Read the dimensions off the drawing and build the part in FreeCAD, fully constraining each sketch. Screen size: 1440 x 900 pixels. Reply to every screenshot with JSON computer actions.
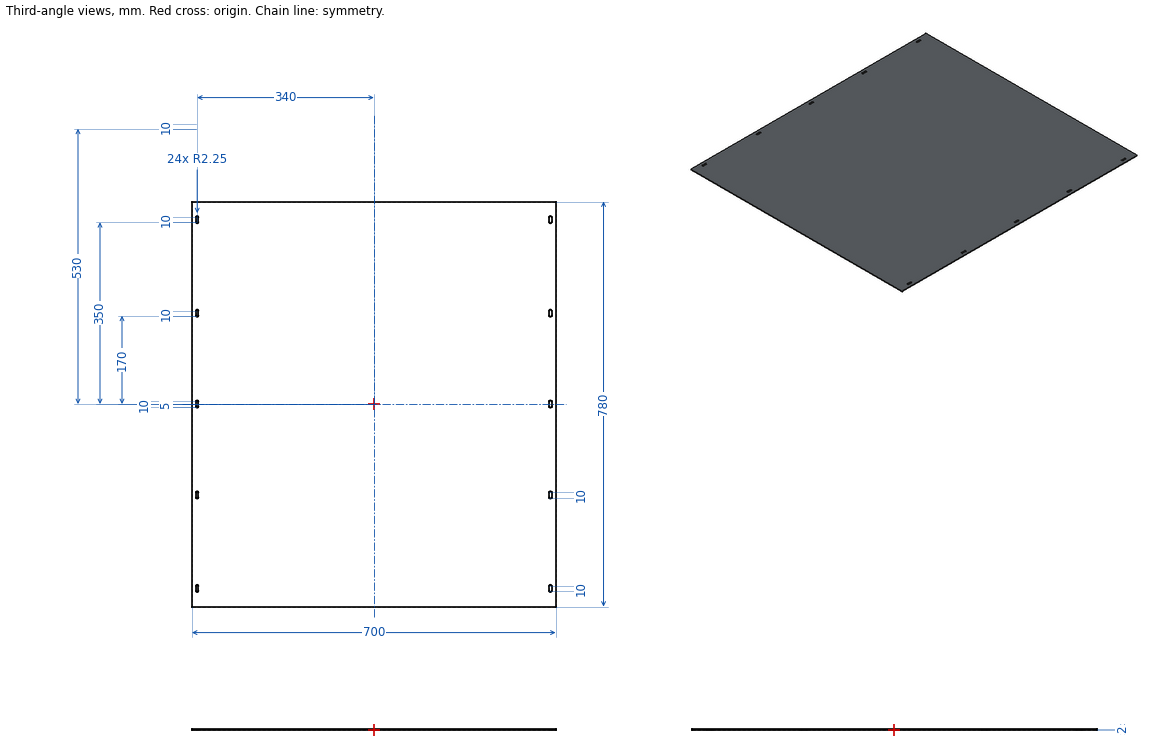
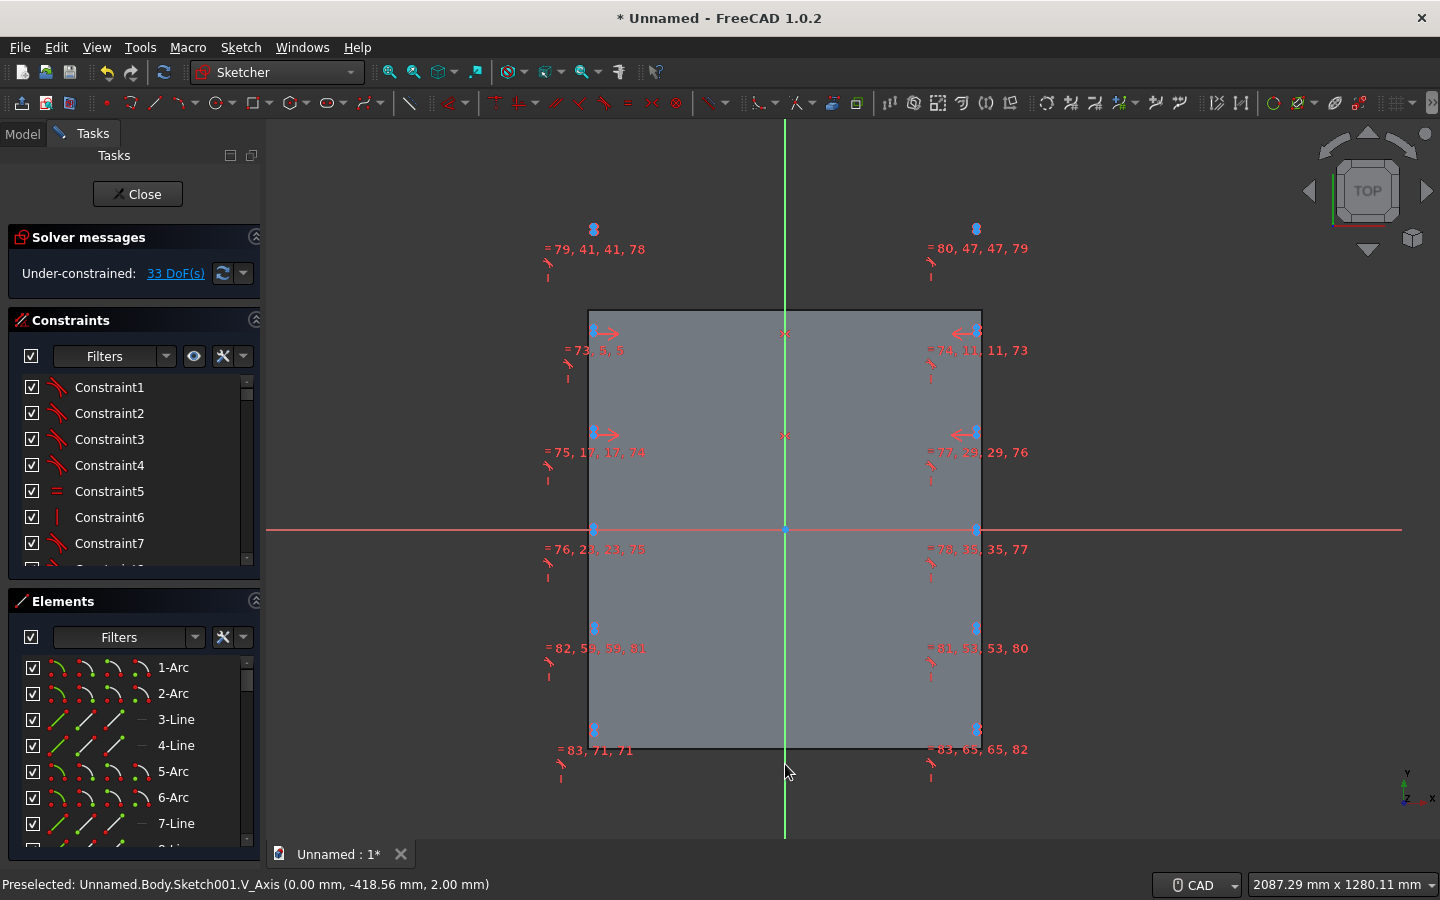
{"action": "scroll", "coordinate": [593, 533], "scroll_direction": "up", "scroll_amount": 12}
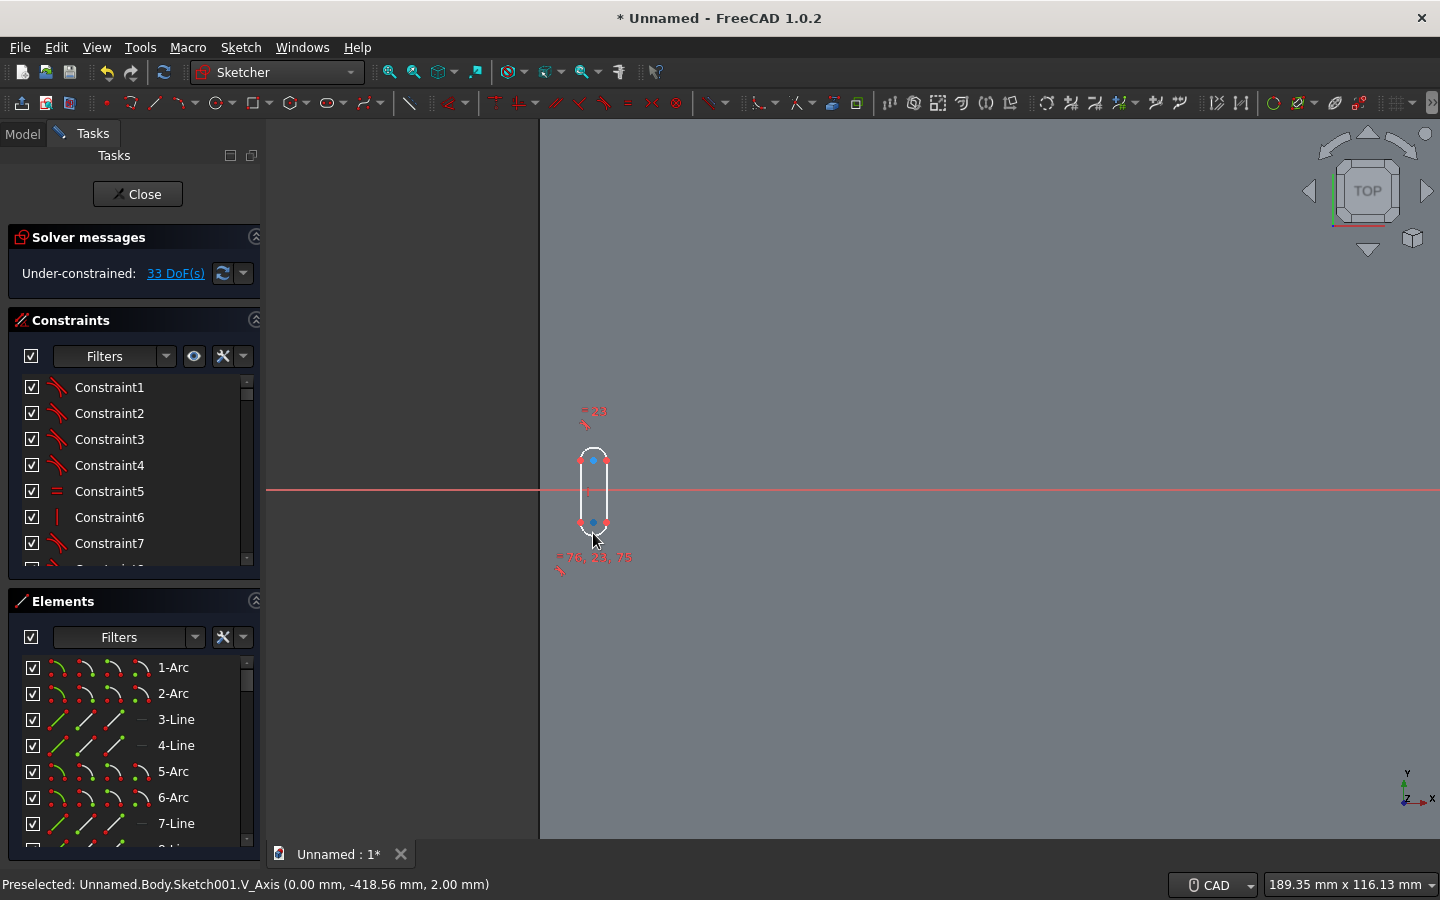
{"action": "left_click", "coordinate": [594, 523]}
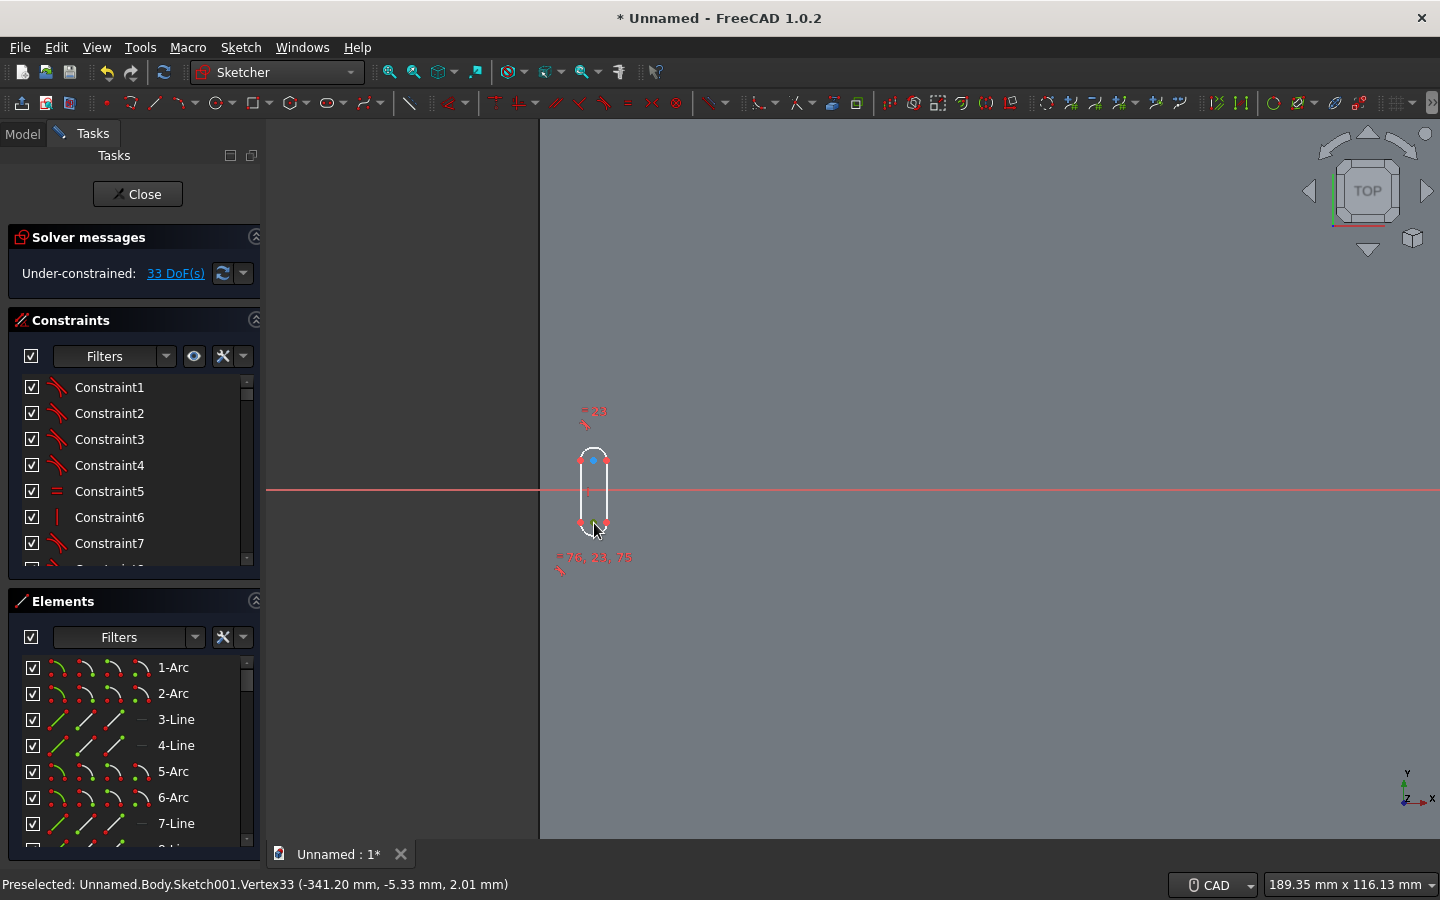
{"action": "scroll", "coordinate": [592, 534], "scroll_direction": "down", "scroll_amount": 12}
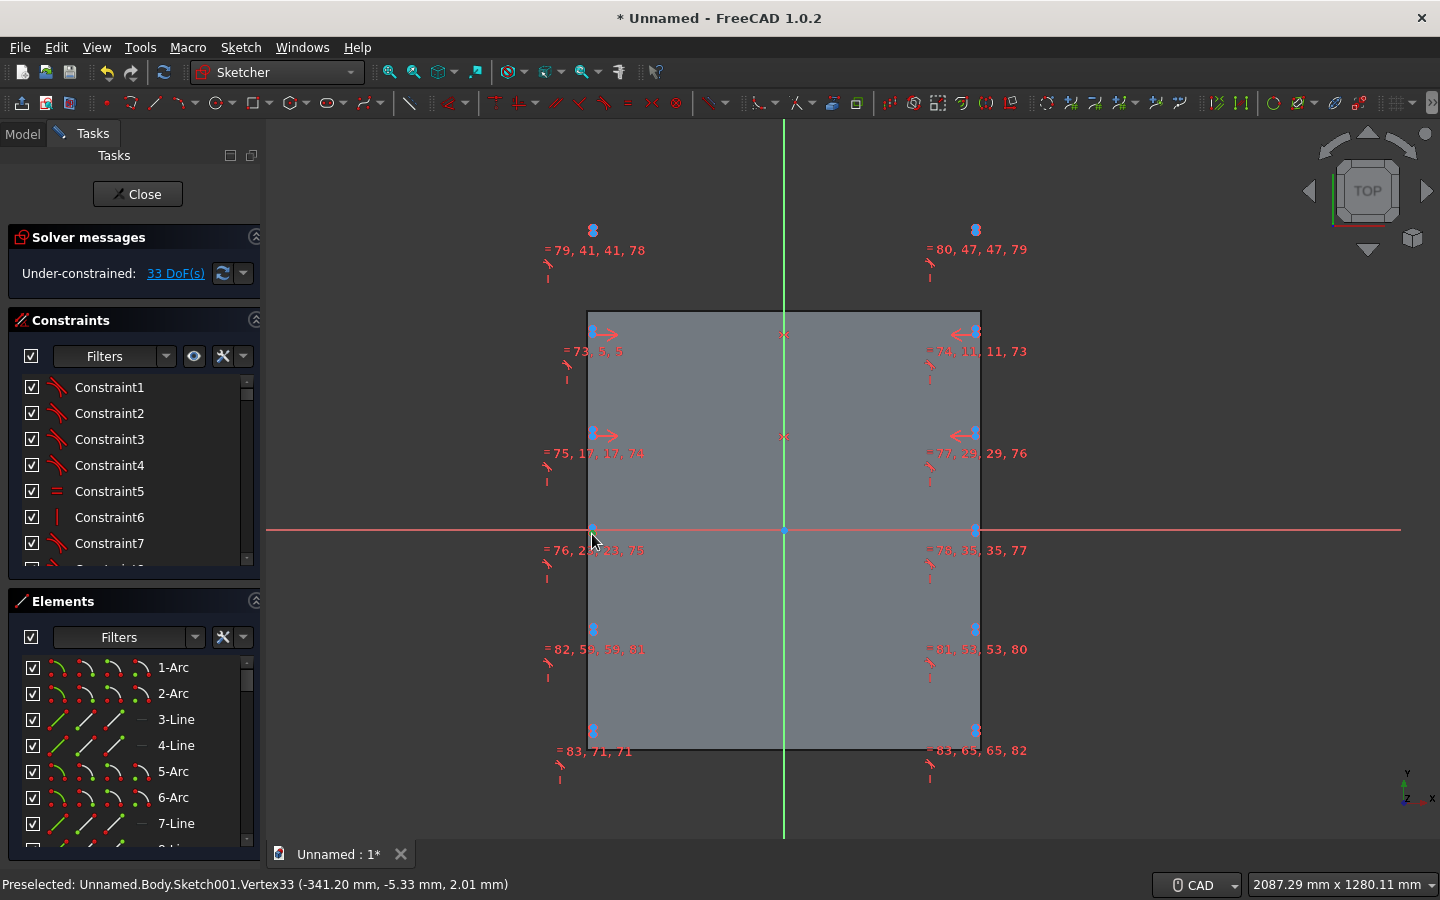
{"action": "scroll", "coordinate": [976, 534], "scroll_direction": "up", "scroll_amount": 12}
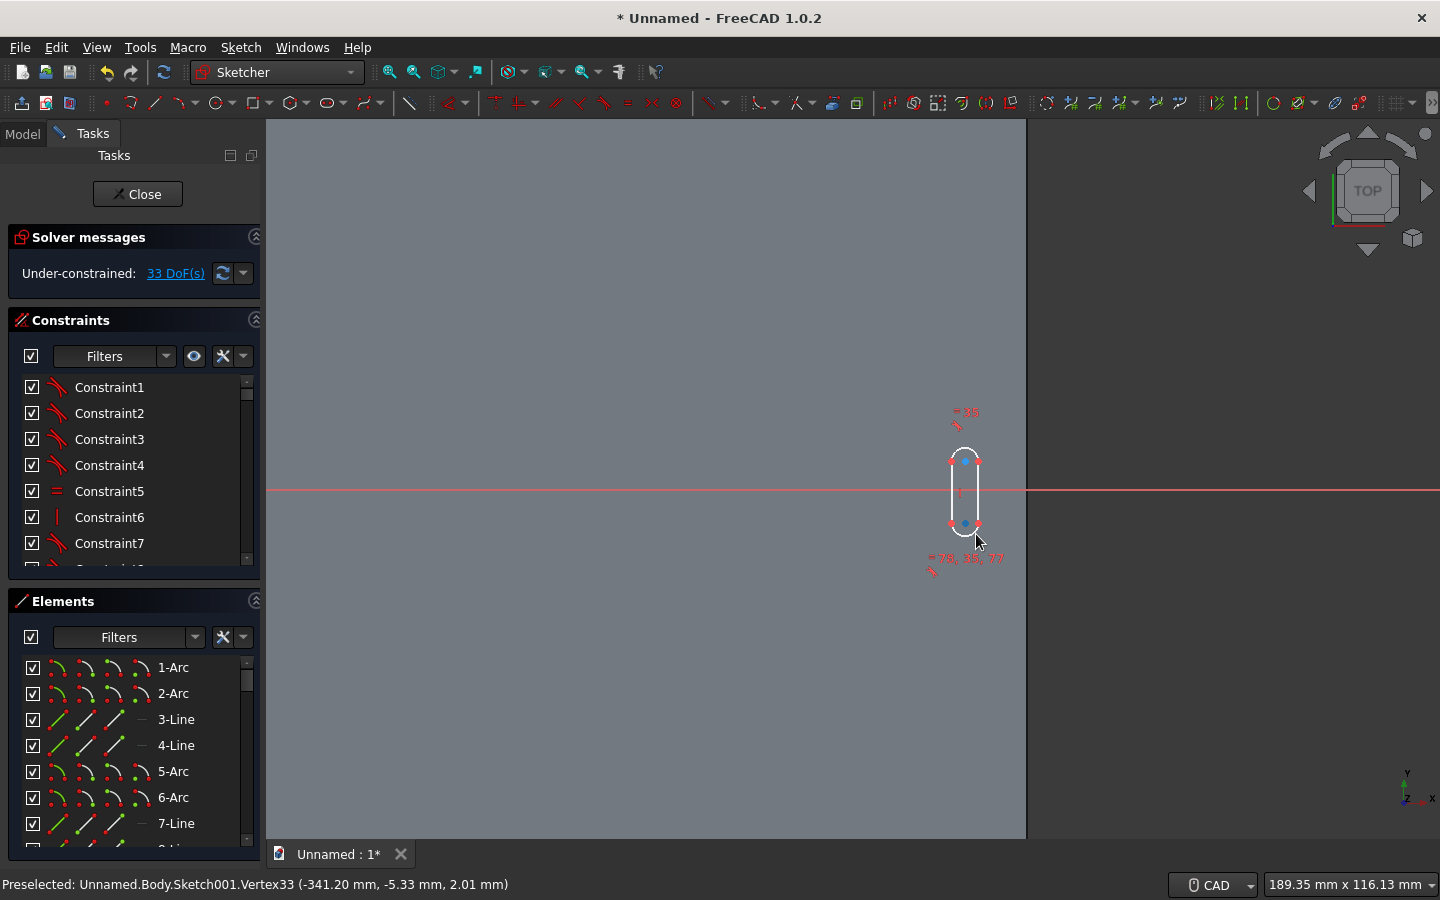
{"action": "left_click", "coordinate": [965, 523]}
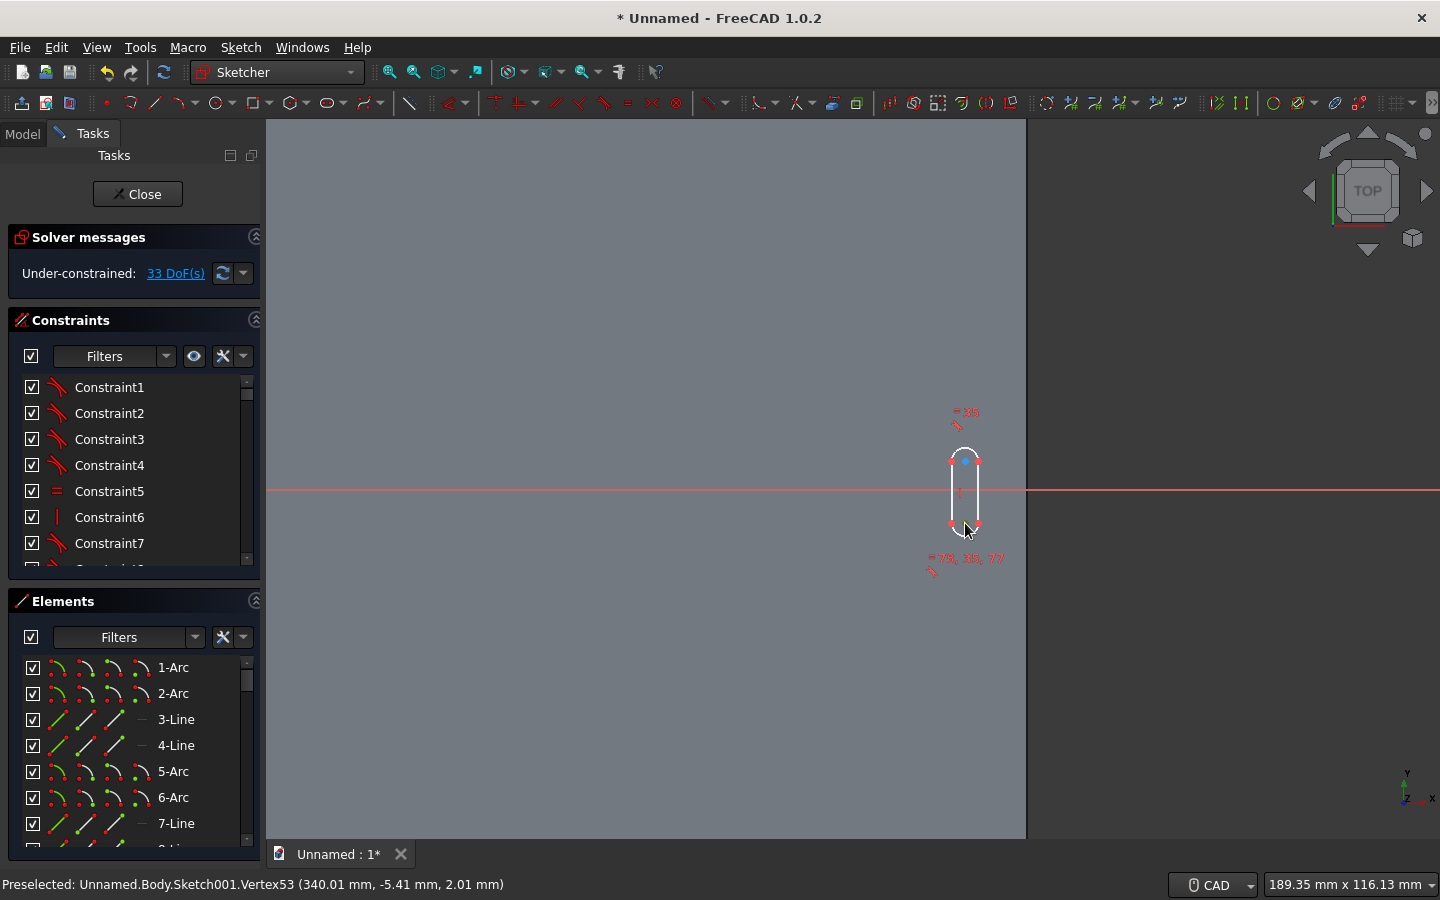
{"action": "scroll", "coordinate": [977, 534], "scroll_direction": "down", "scroll_amount": 12}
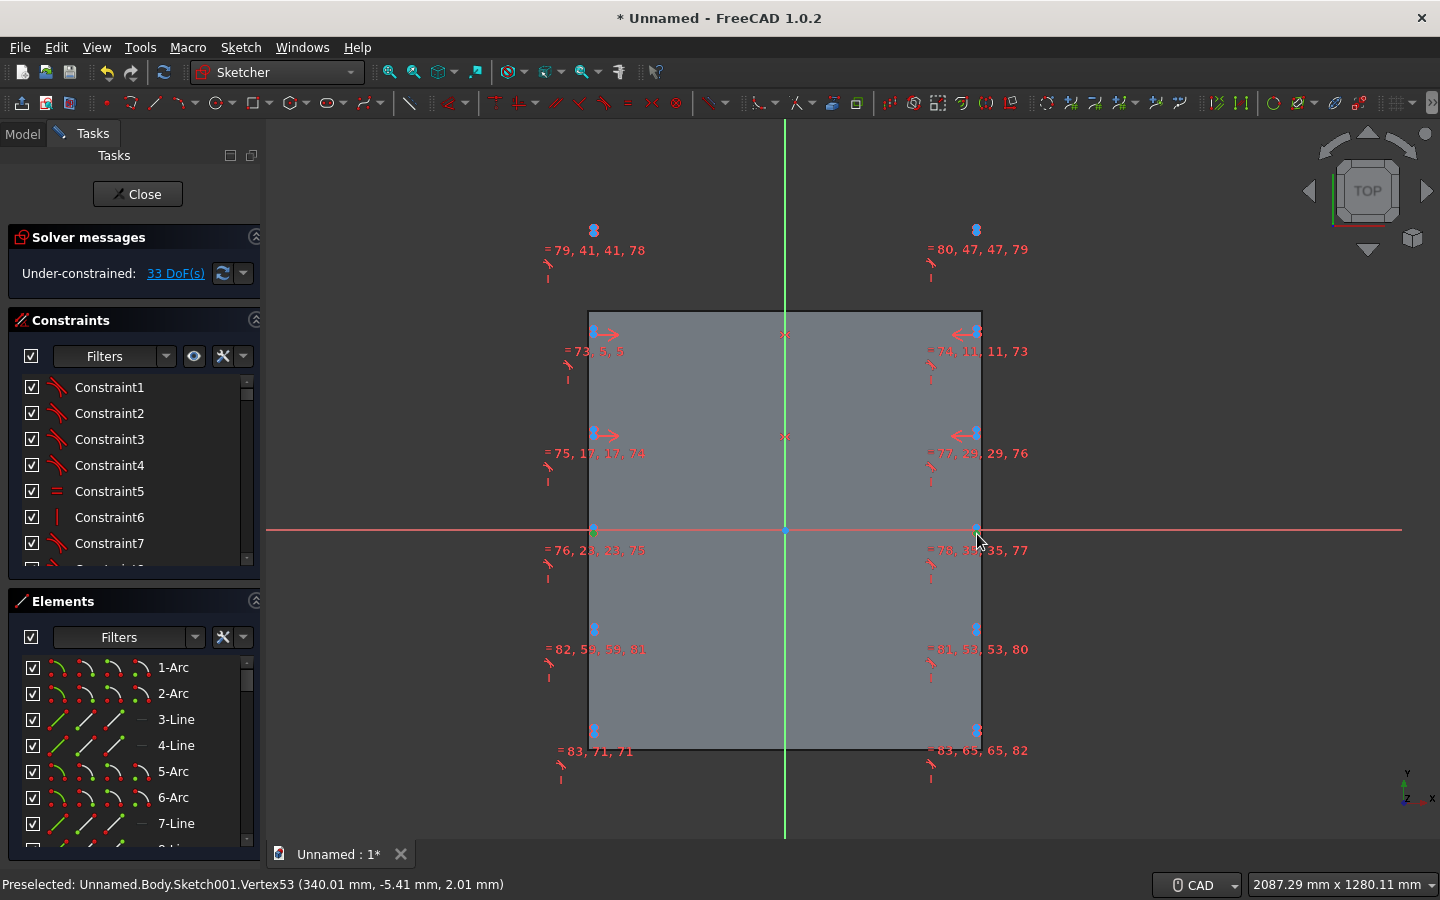
{"action": "left_click", "coordinate": [785, 764]}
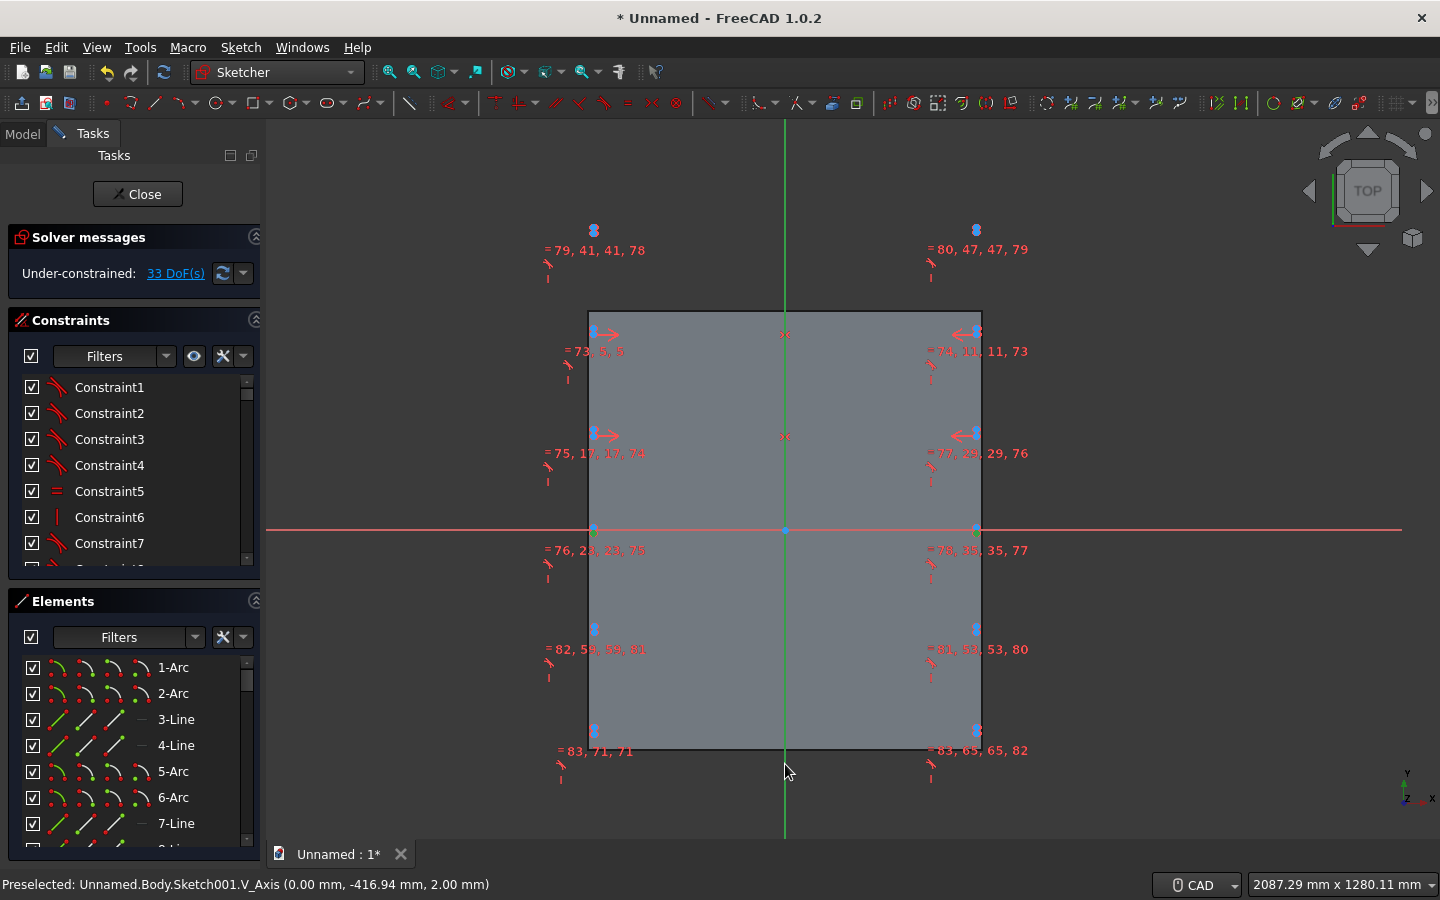
{"action": "left_click", "coordinate": [652, 104]}